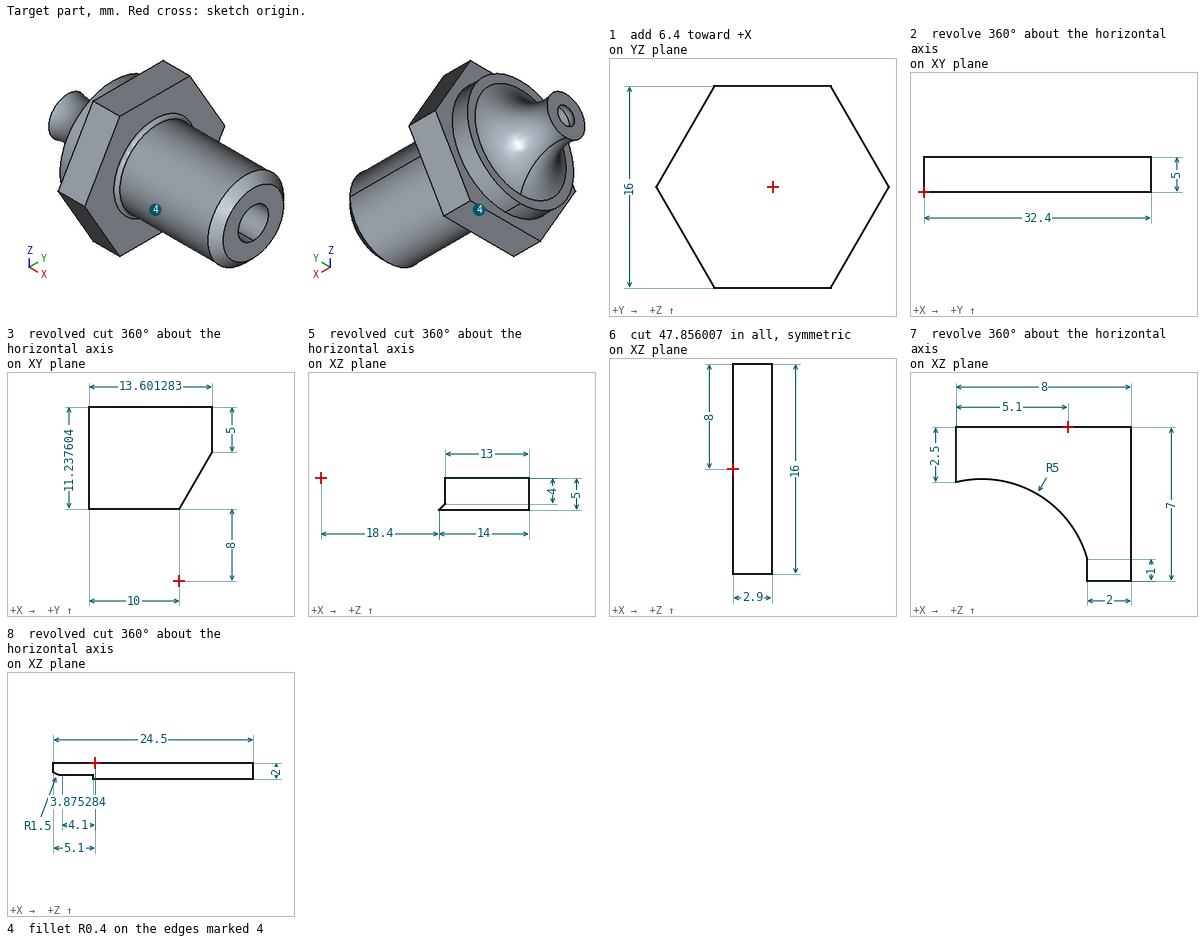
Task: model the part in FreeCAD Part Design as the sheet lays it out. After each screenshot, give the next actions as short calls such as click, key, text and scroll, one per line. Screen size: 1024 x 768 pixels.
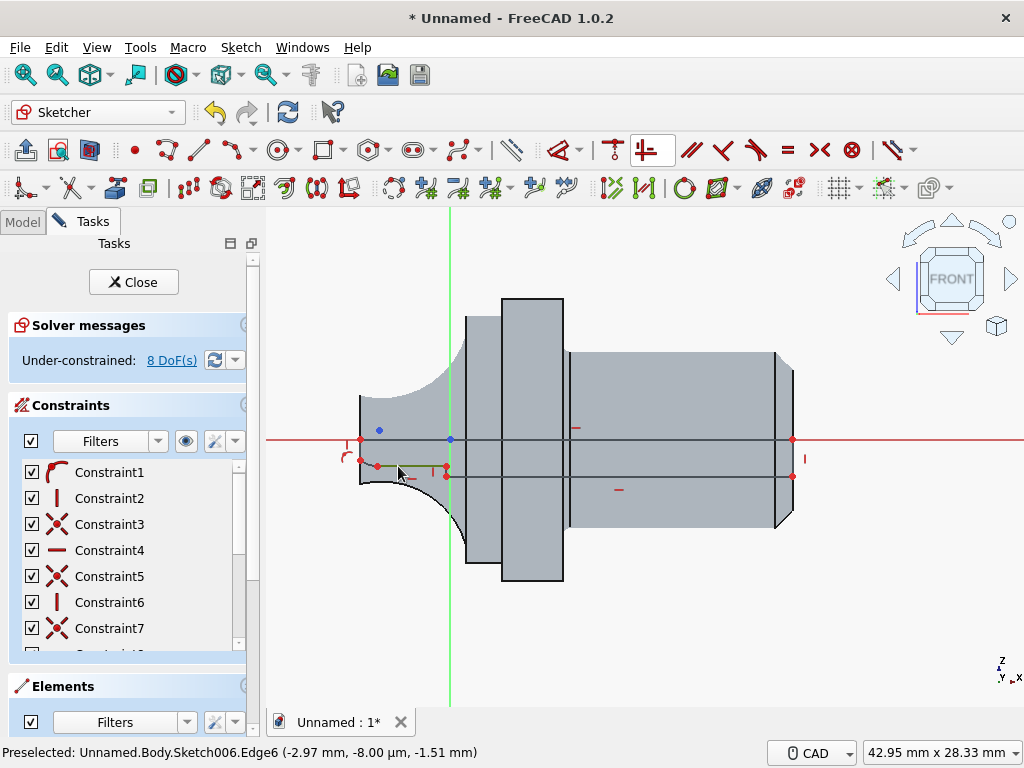
scroll(369, 465, up, 2)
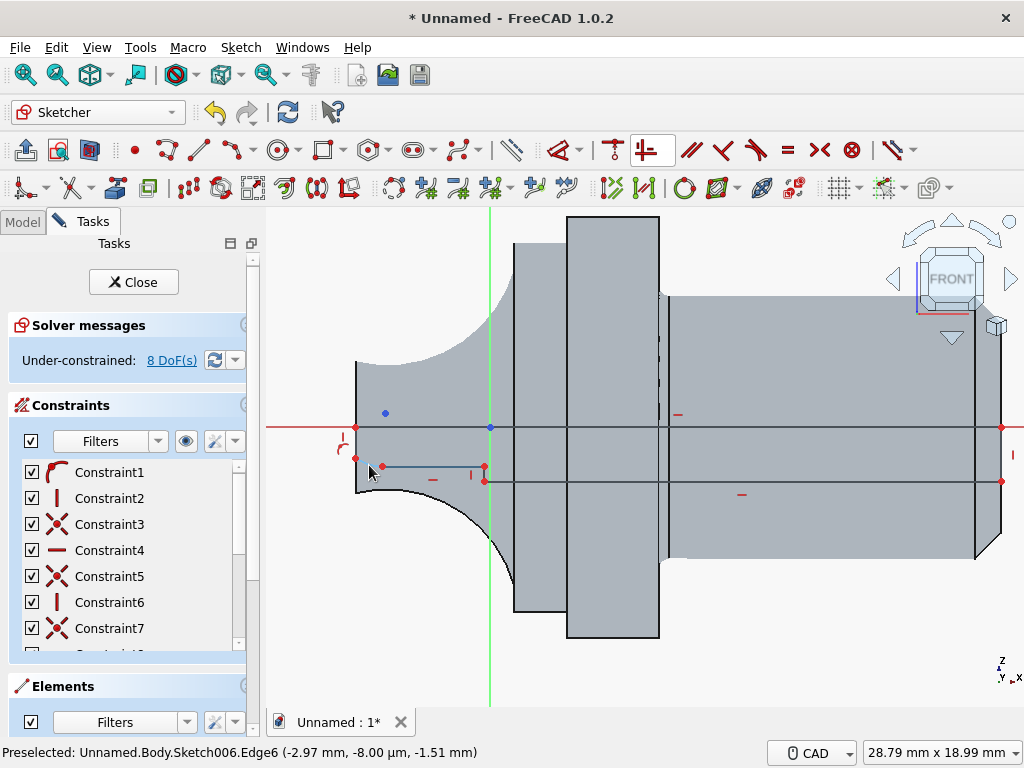
click(369, 464)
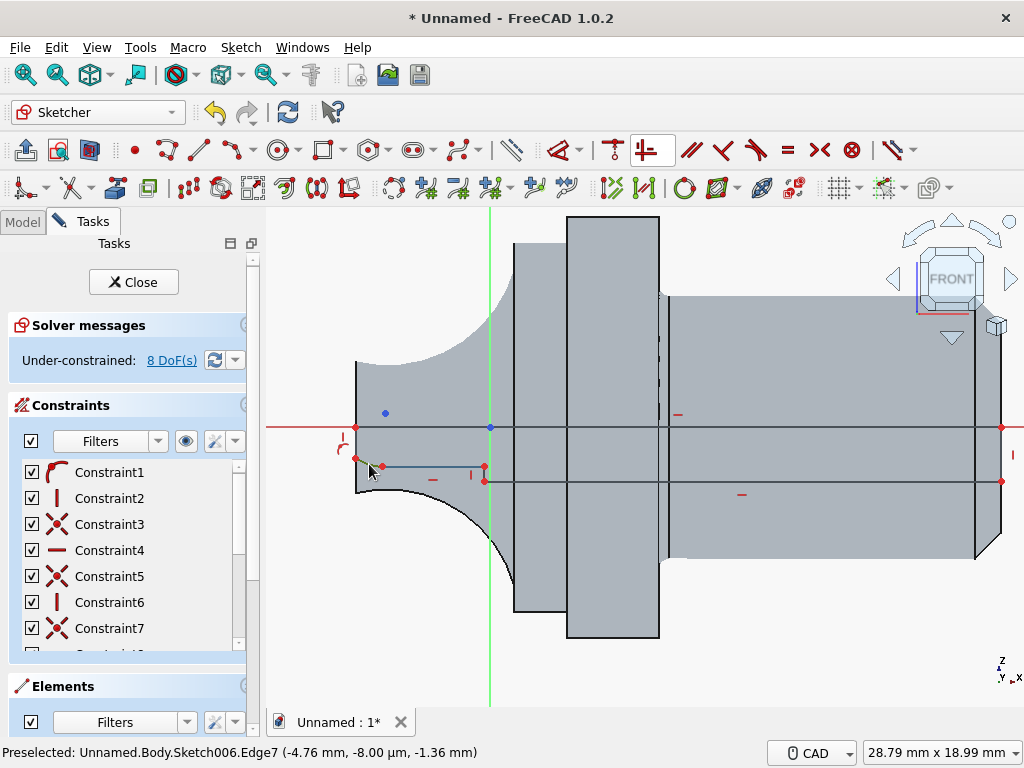
click(756, 150)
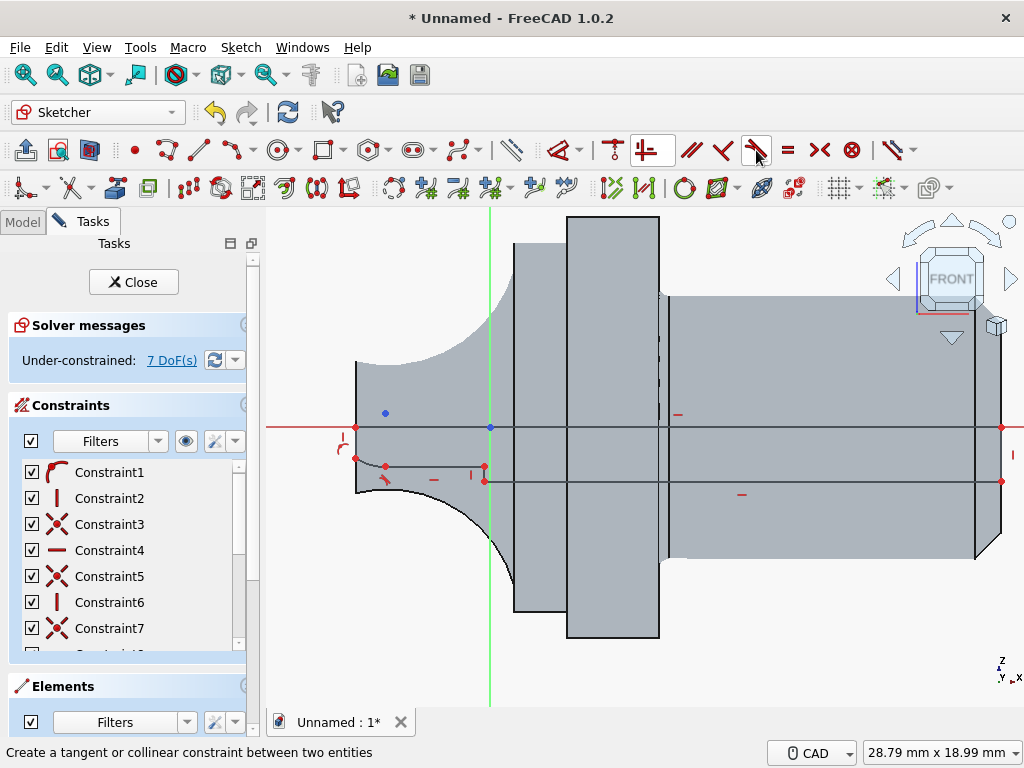
click(385, 414)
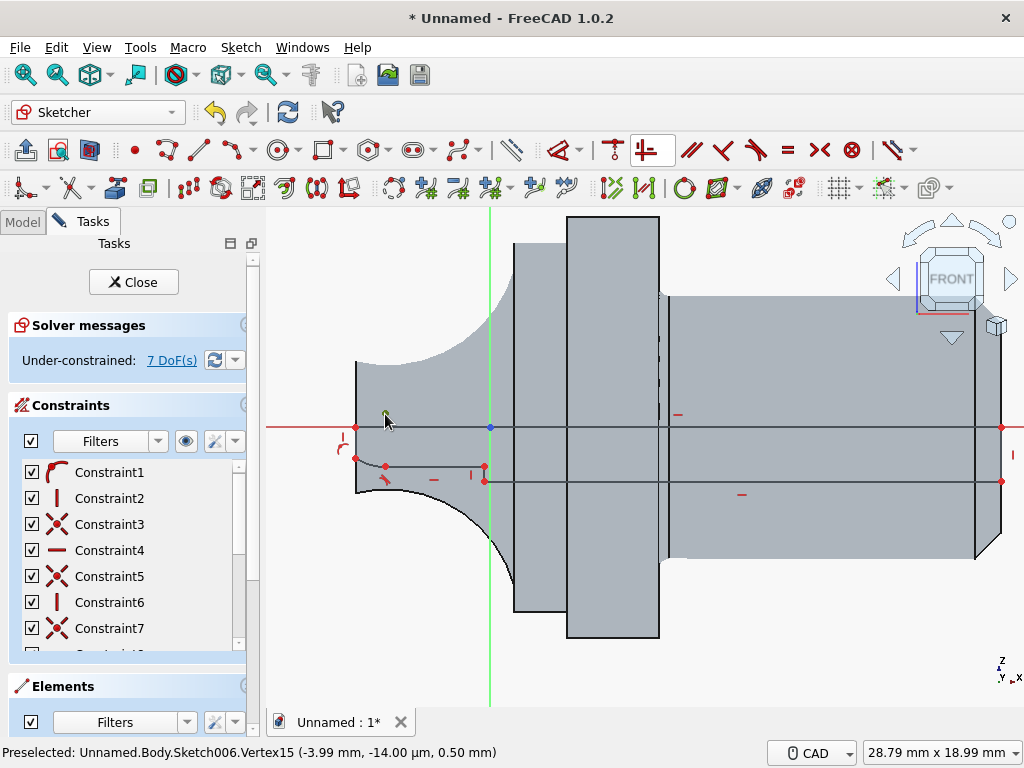
click(334, 427)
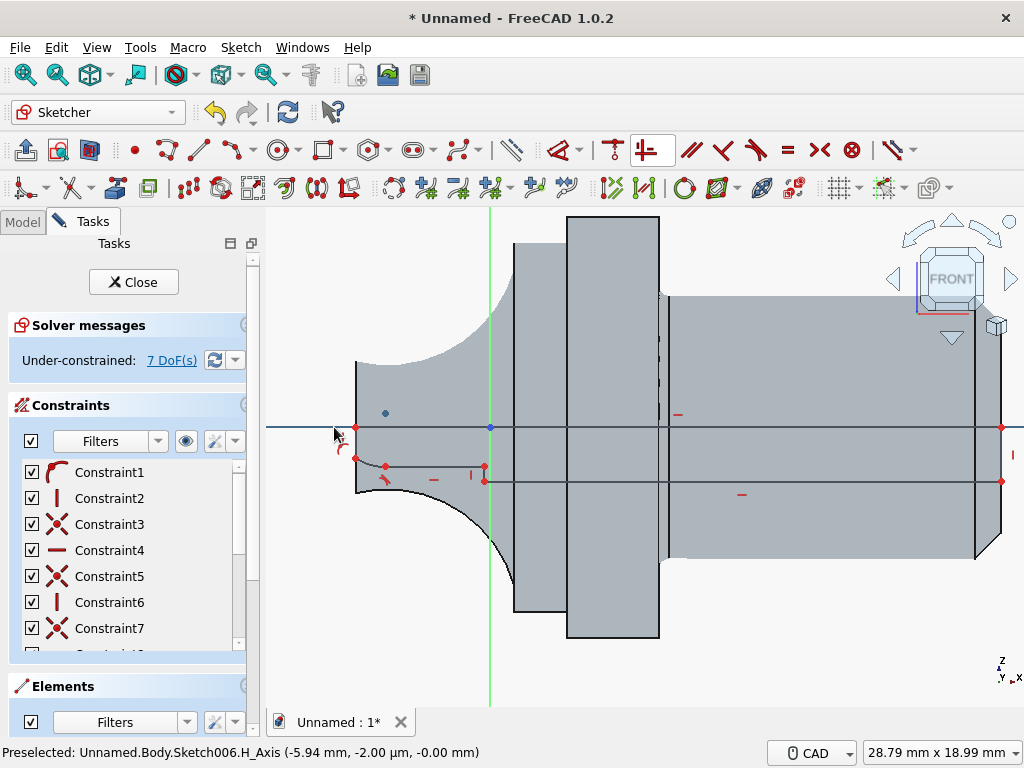
click(614, 150)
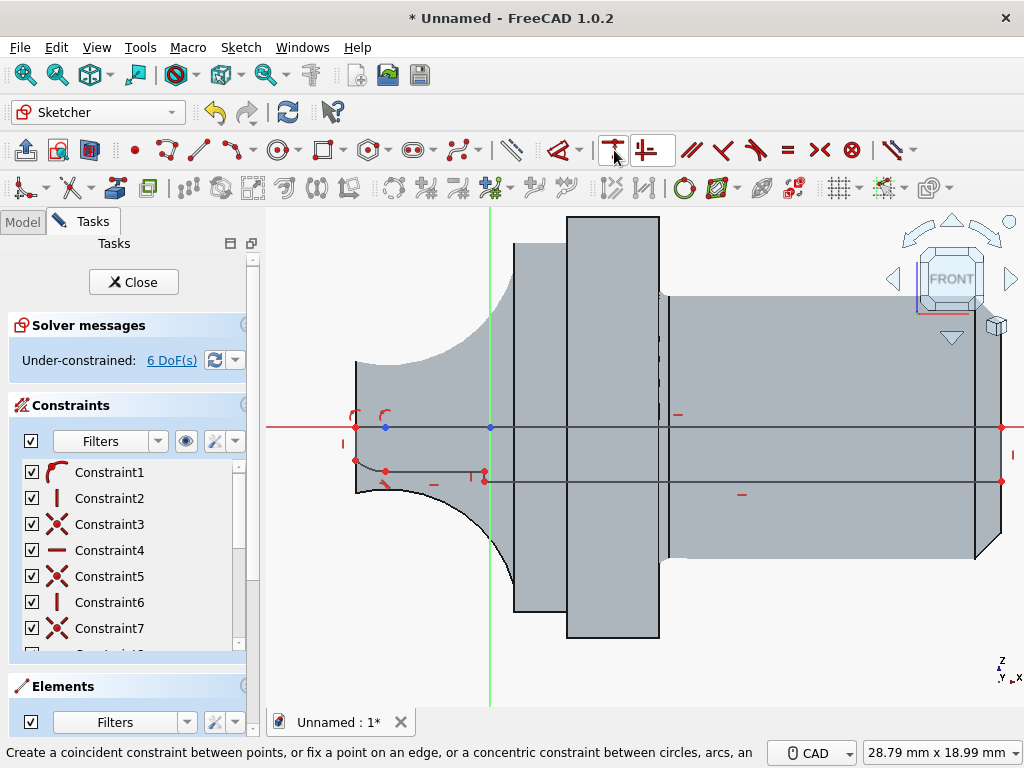
click(558, 150)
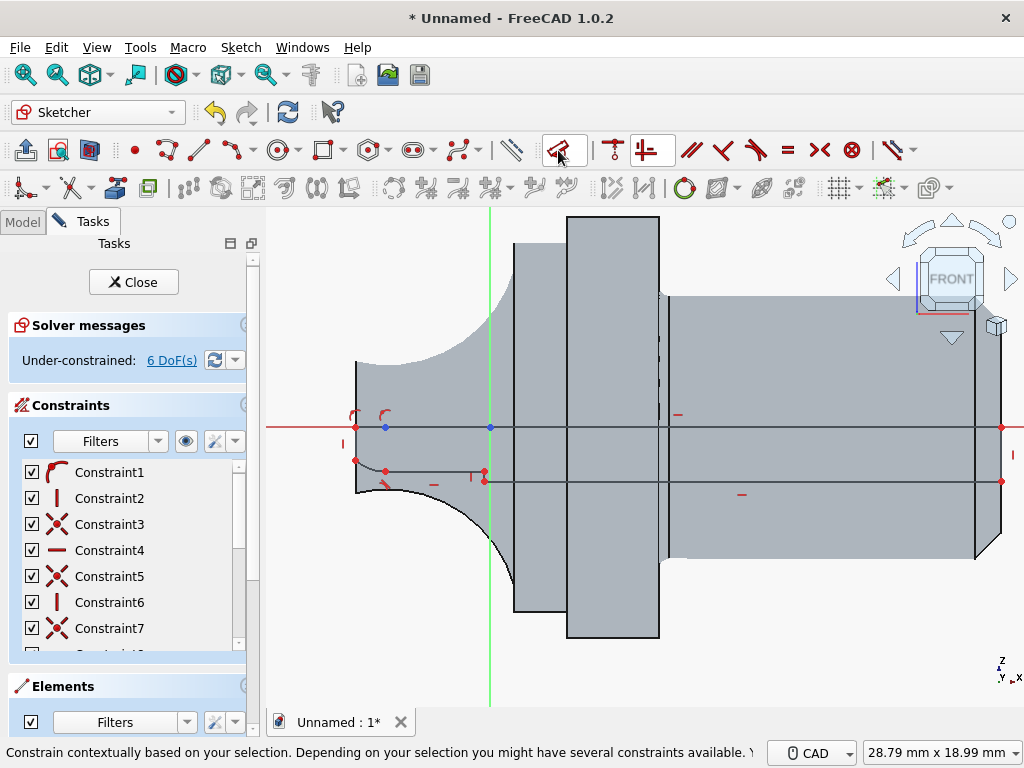
scroll(364, 466, up, 2)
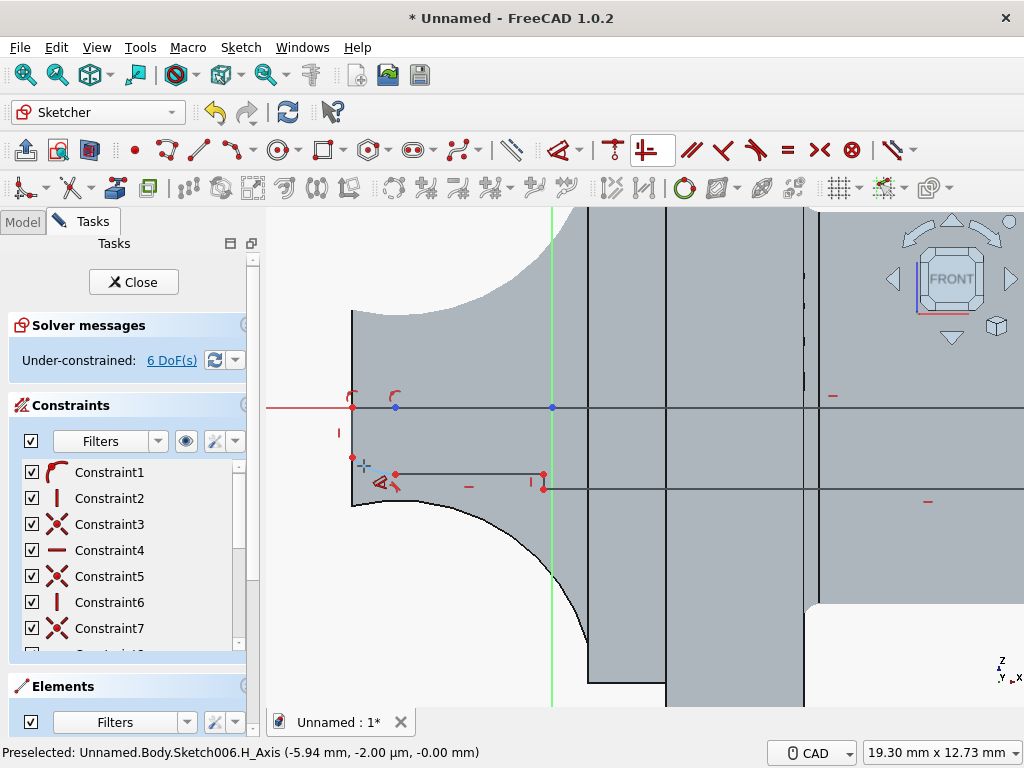
click(364, 466)
click(349, 494)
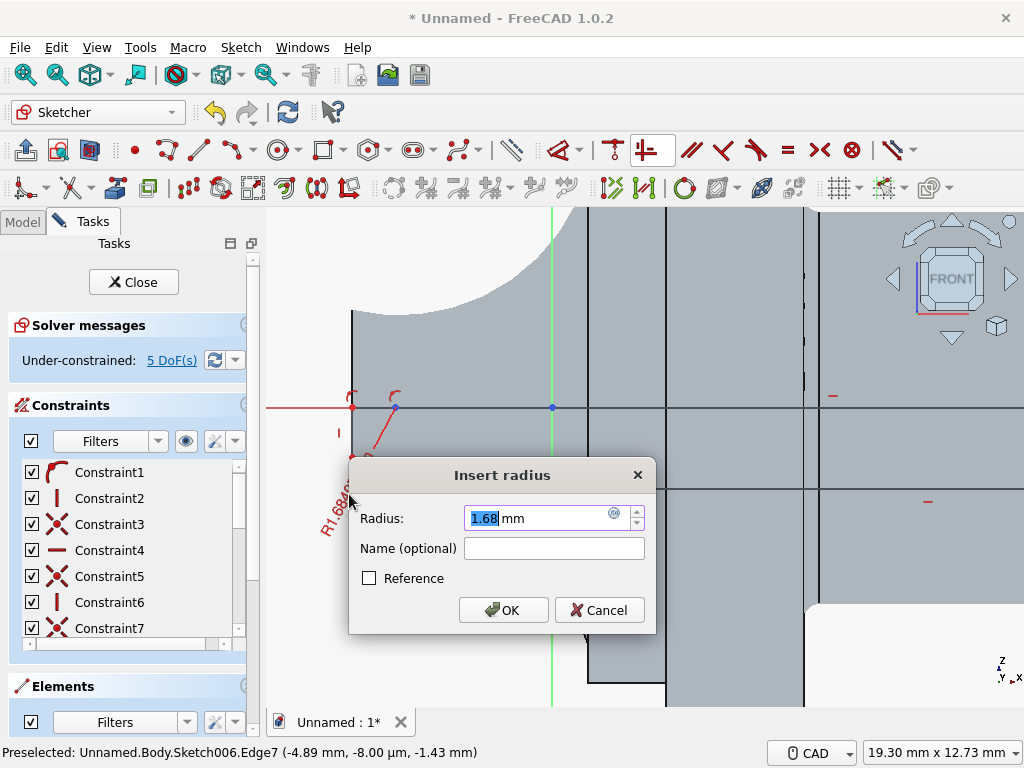
text(1.5)
key(Return)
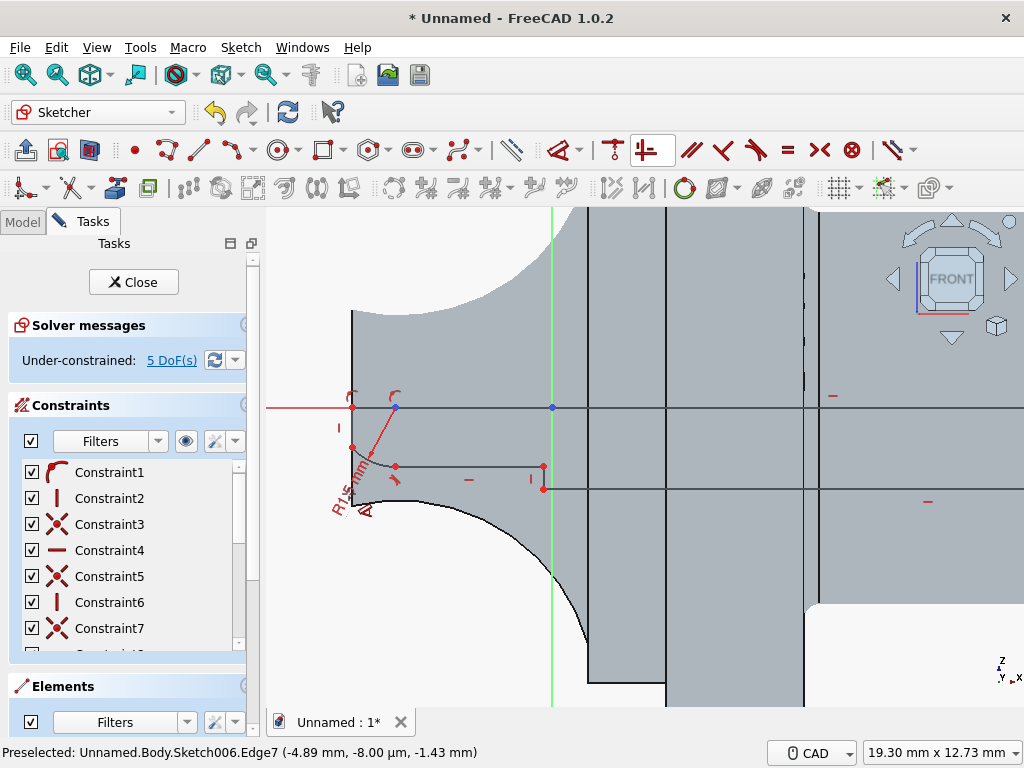
scroll(367, 465, down, 4)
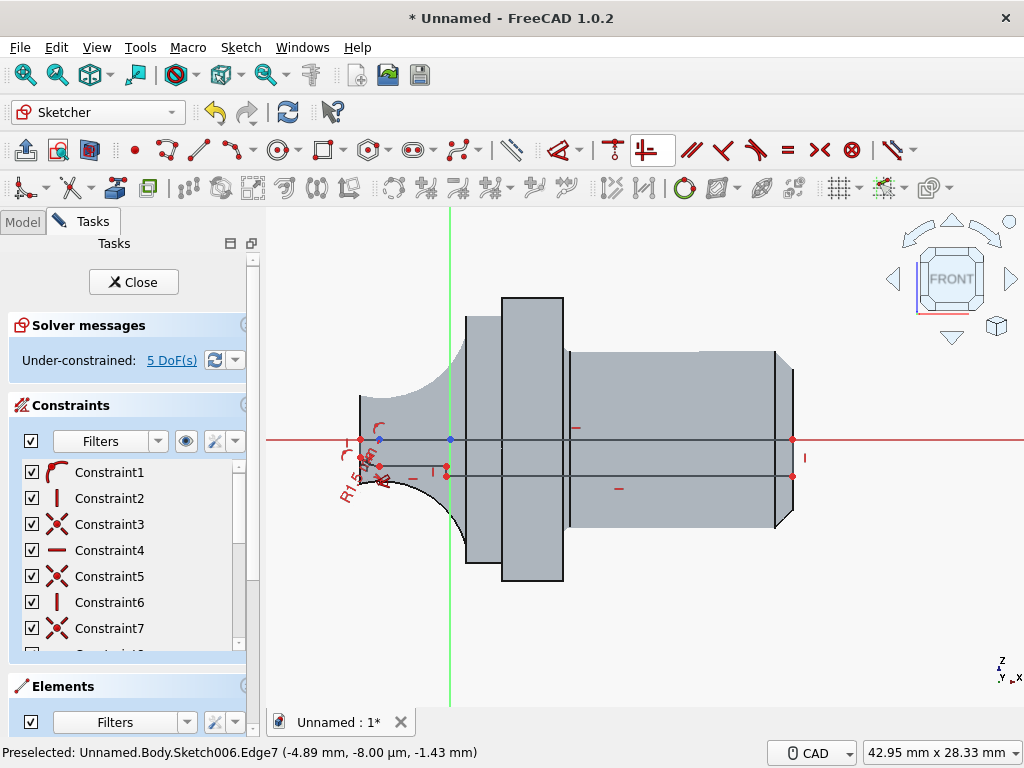
scroll(793, 451, up, 2)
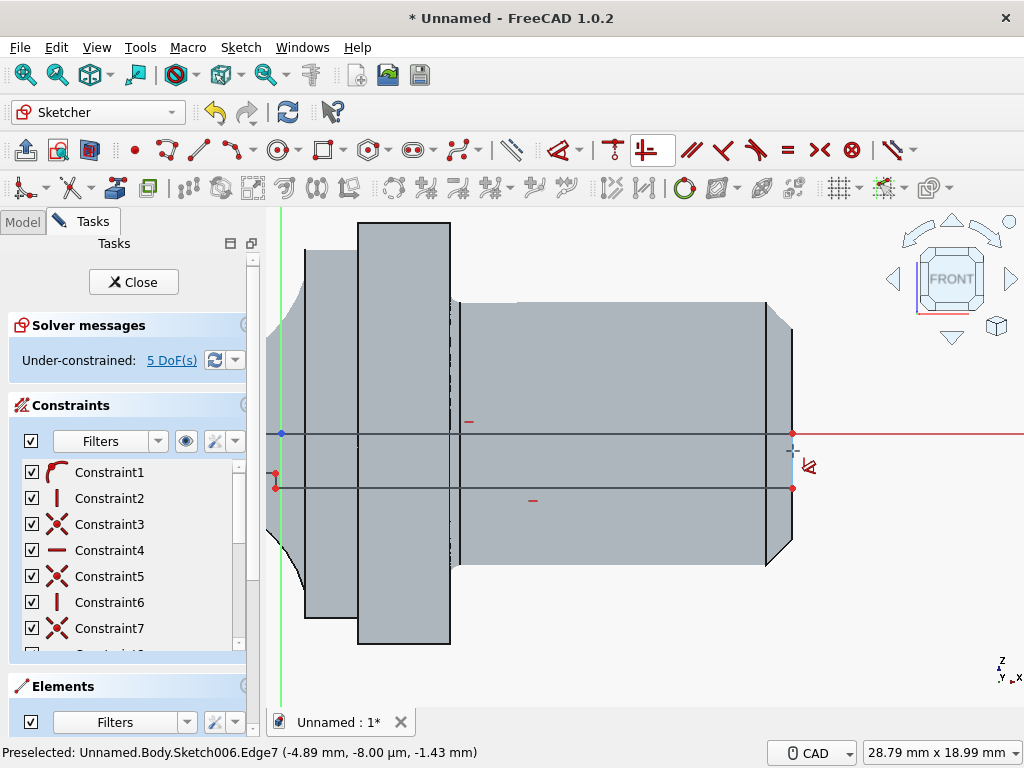
click(792, 450)
click(826, 461)